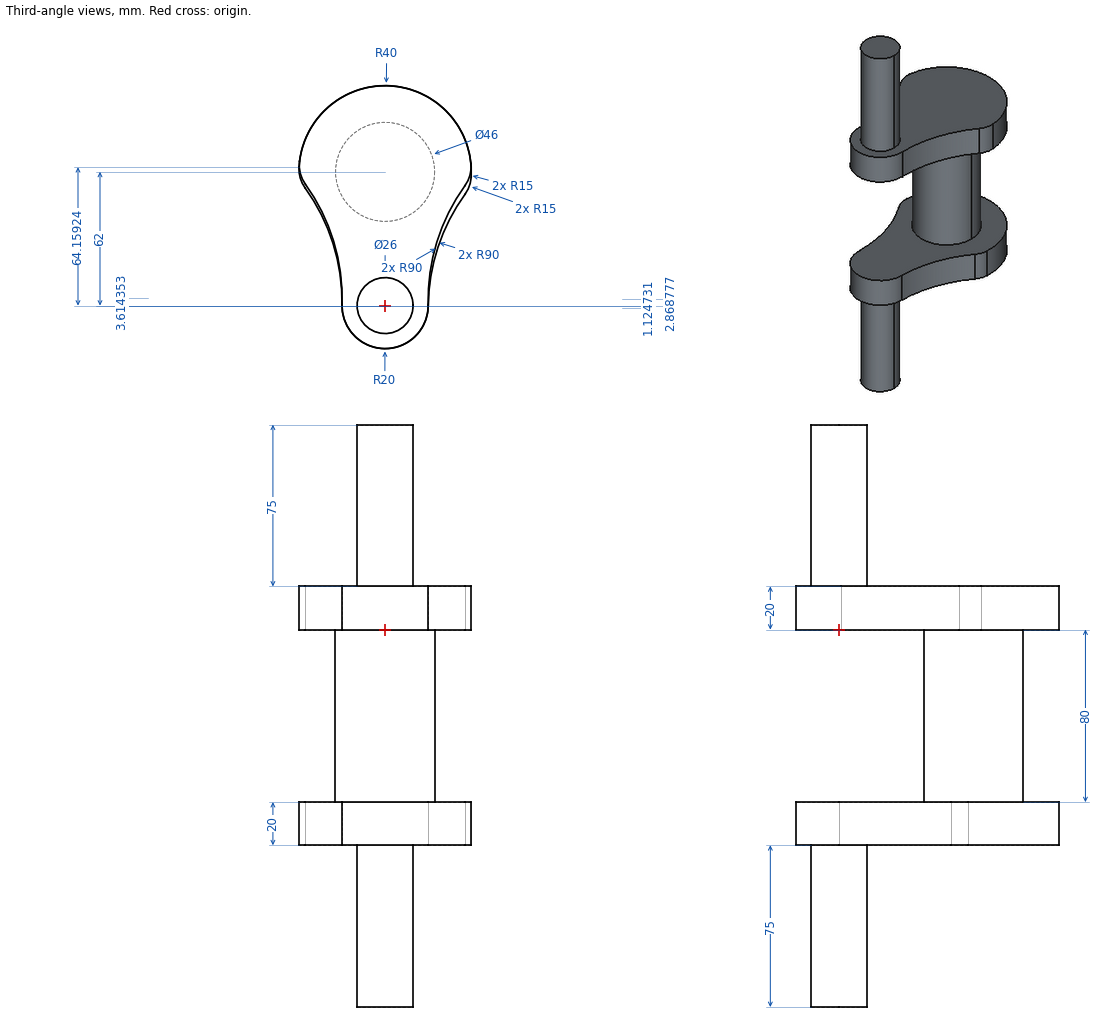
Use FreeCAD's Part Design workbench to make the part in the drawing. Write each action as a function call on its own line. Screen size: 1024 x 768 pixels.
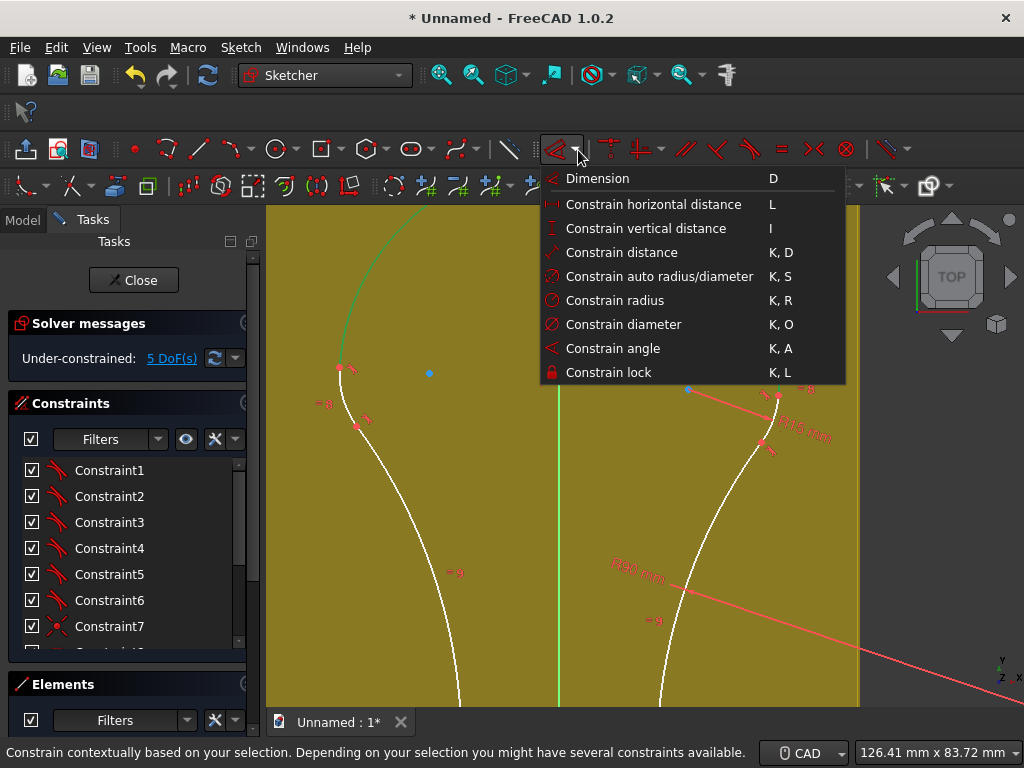
click(693, 300)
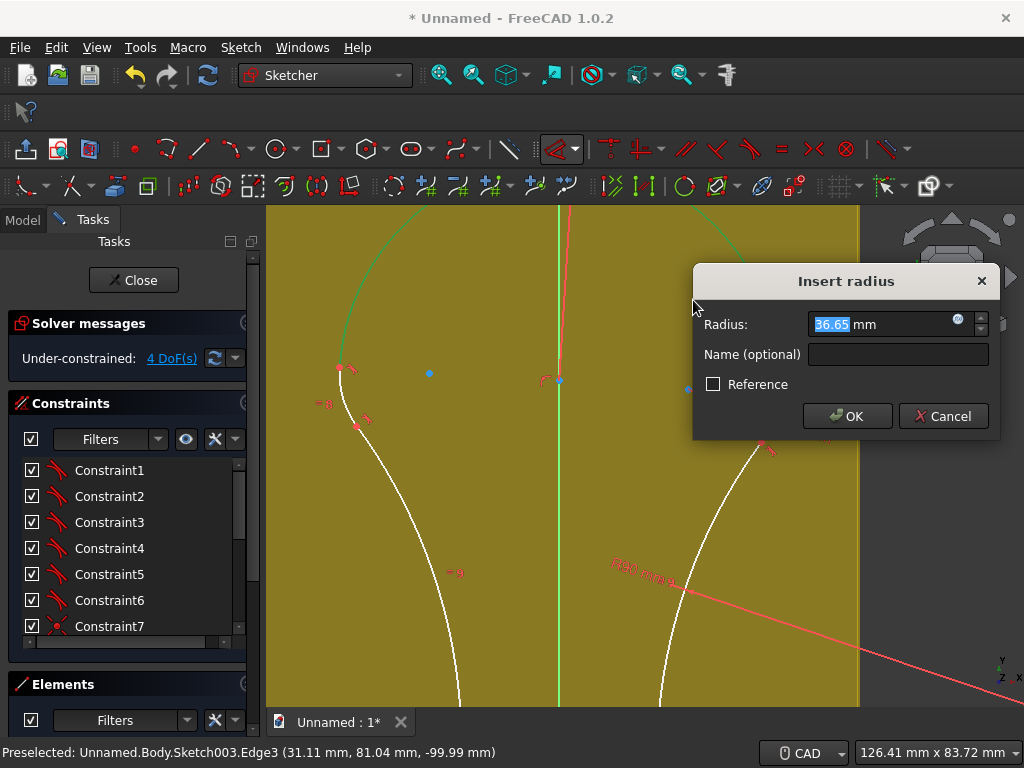
text(40)
key(Return)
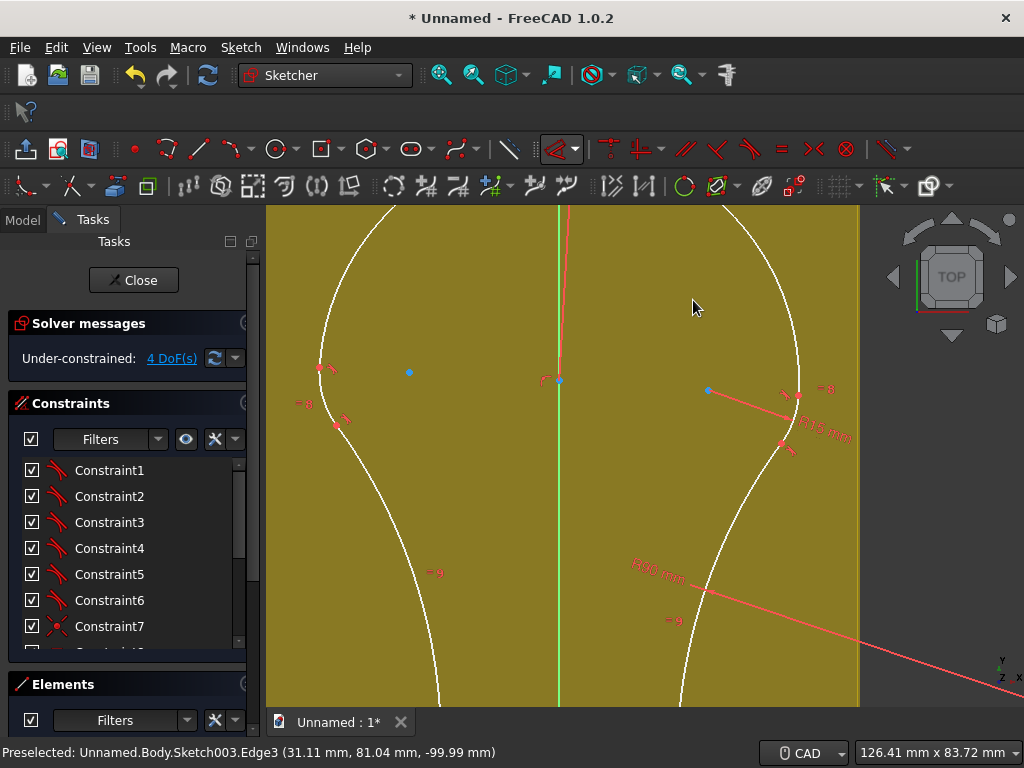
scroll(591, 416, down, 4)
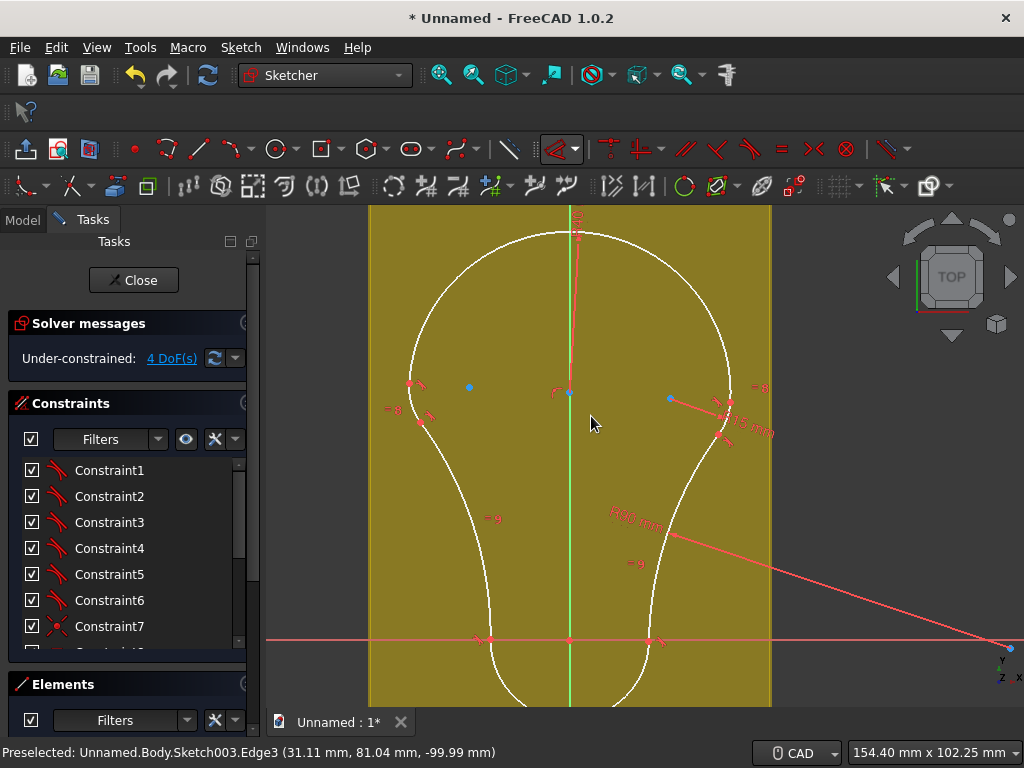
click(545, 609)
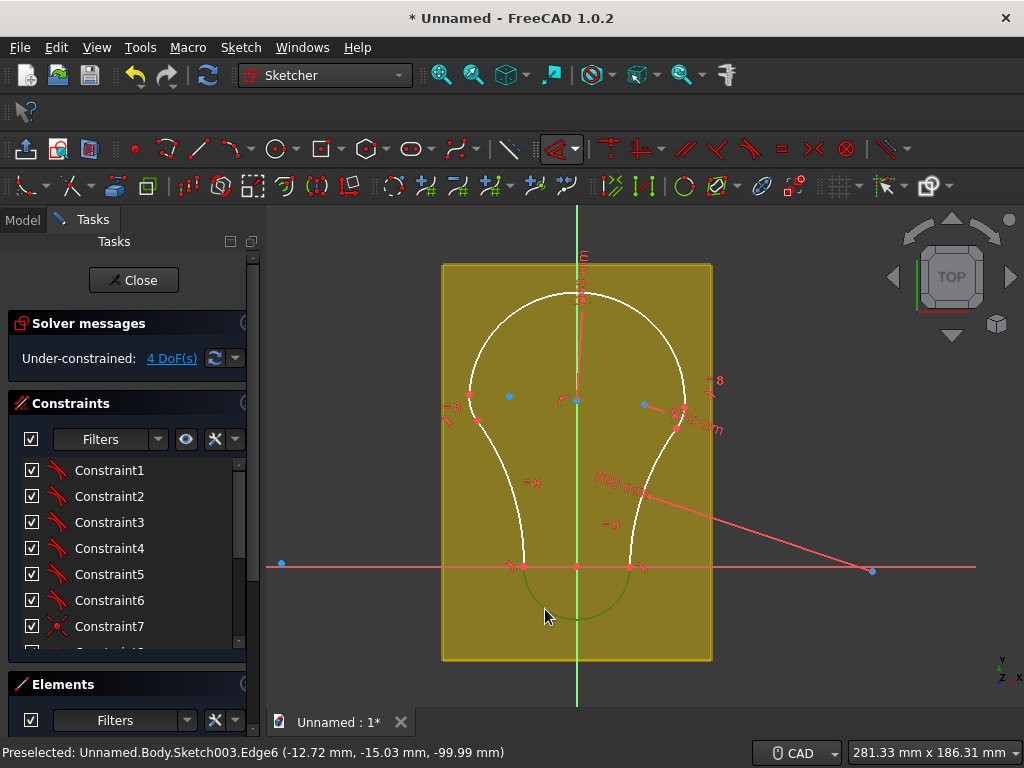
key(k)
key(r)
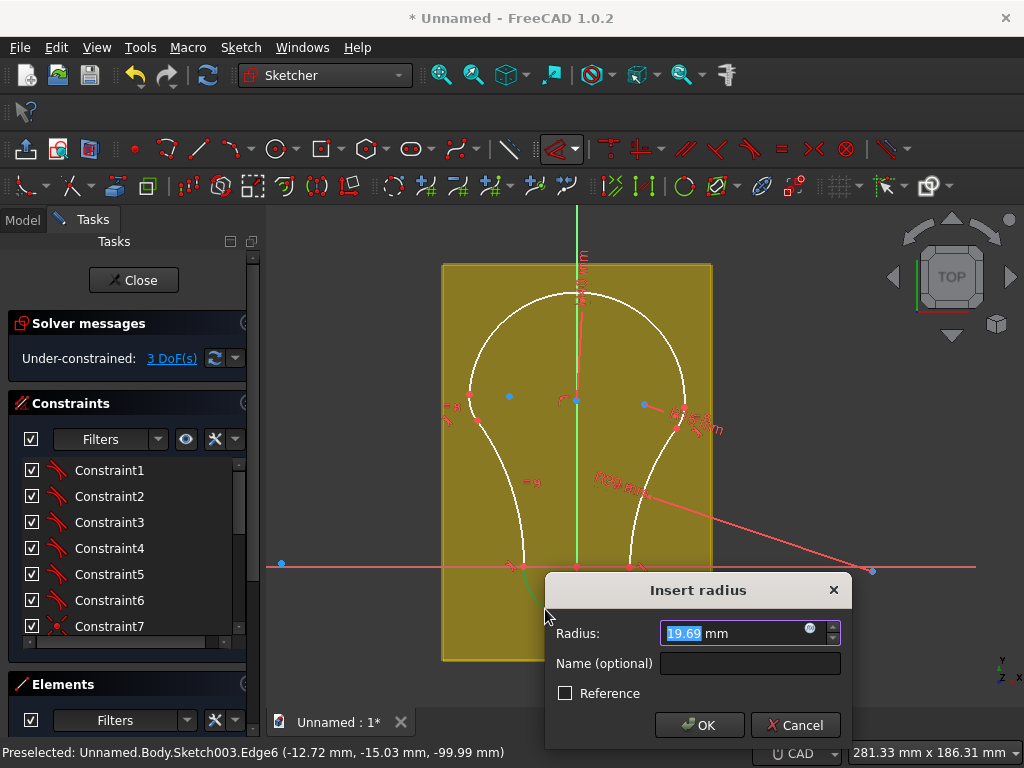
text(20)
key(Return)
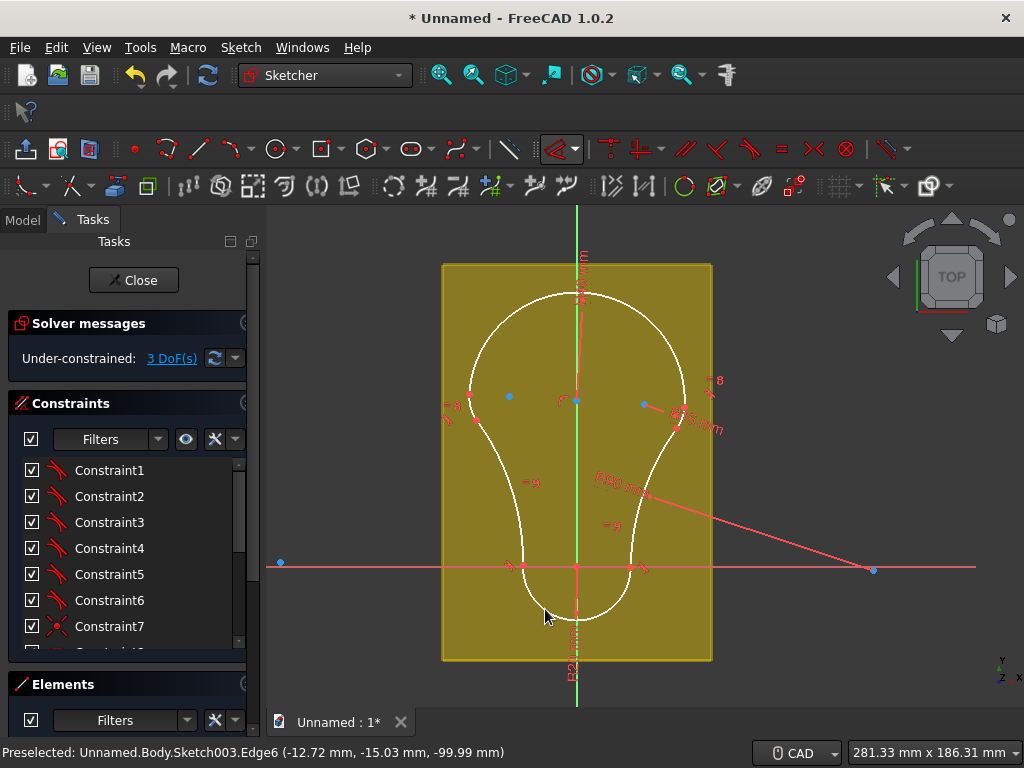
click(577, 400)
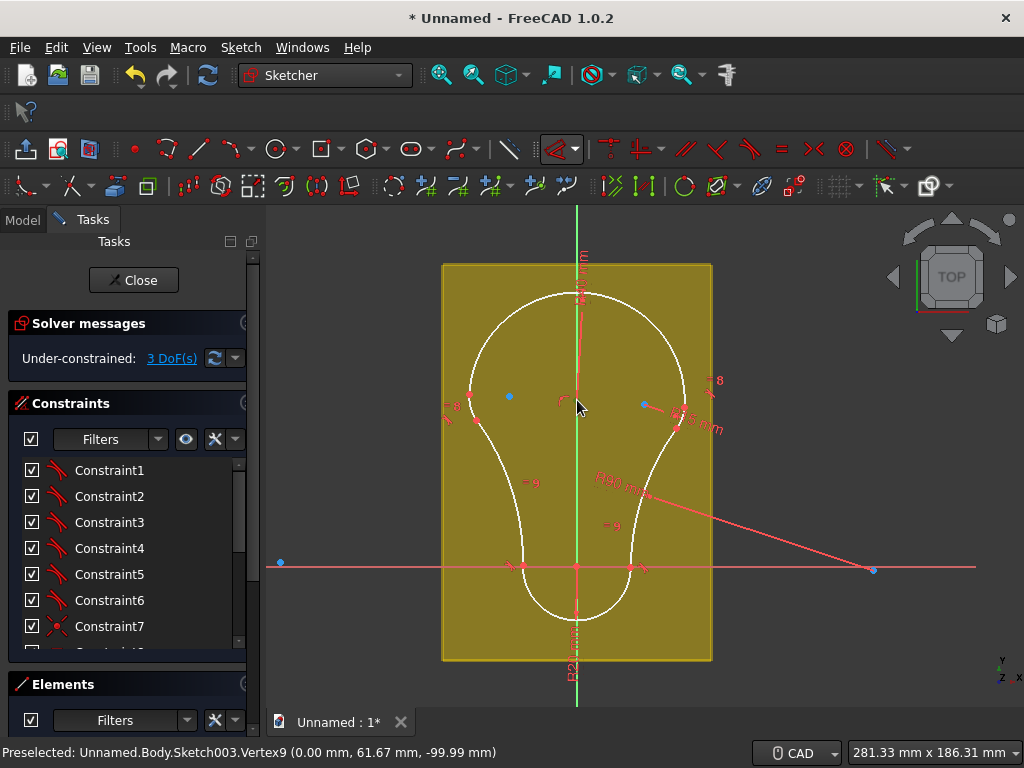
key(i)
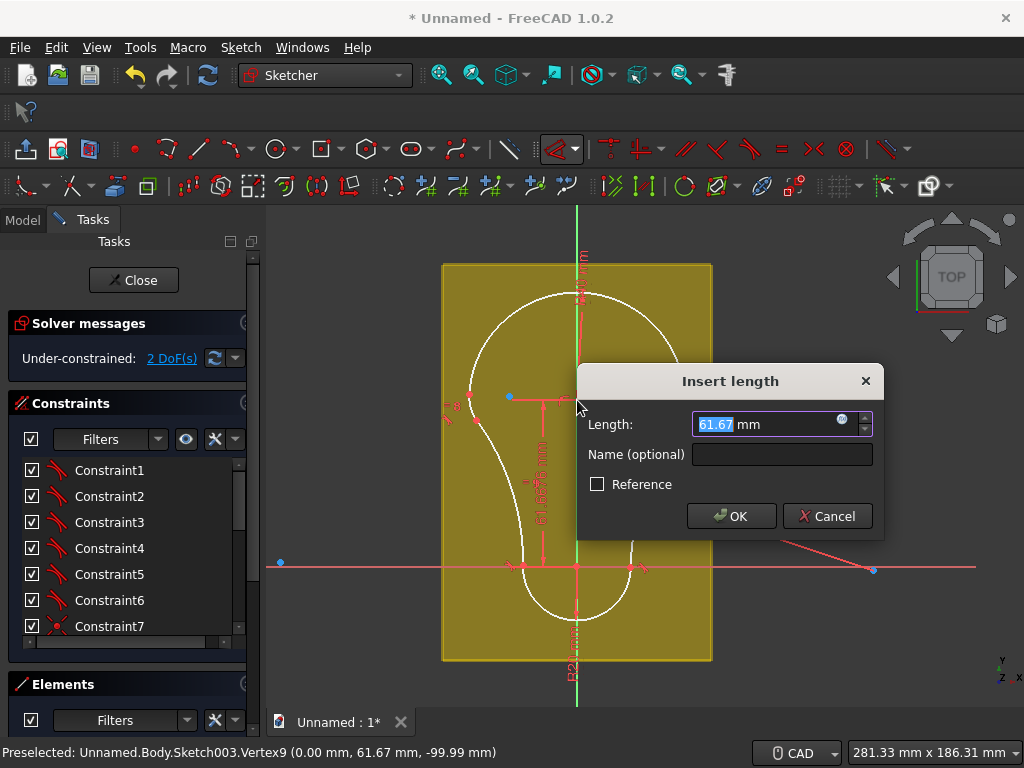
text(62)
key(Return)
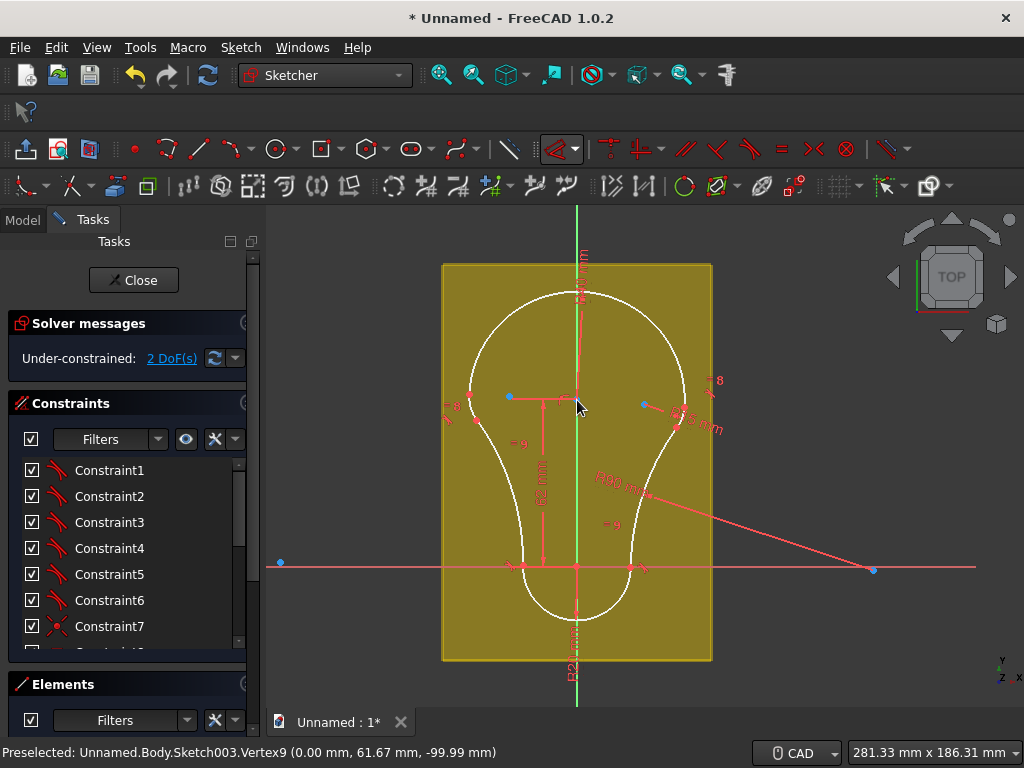
click(469, 395)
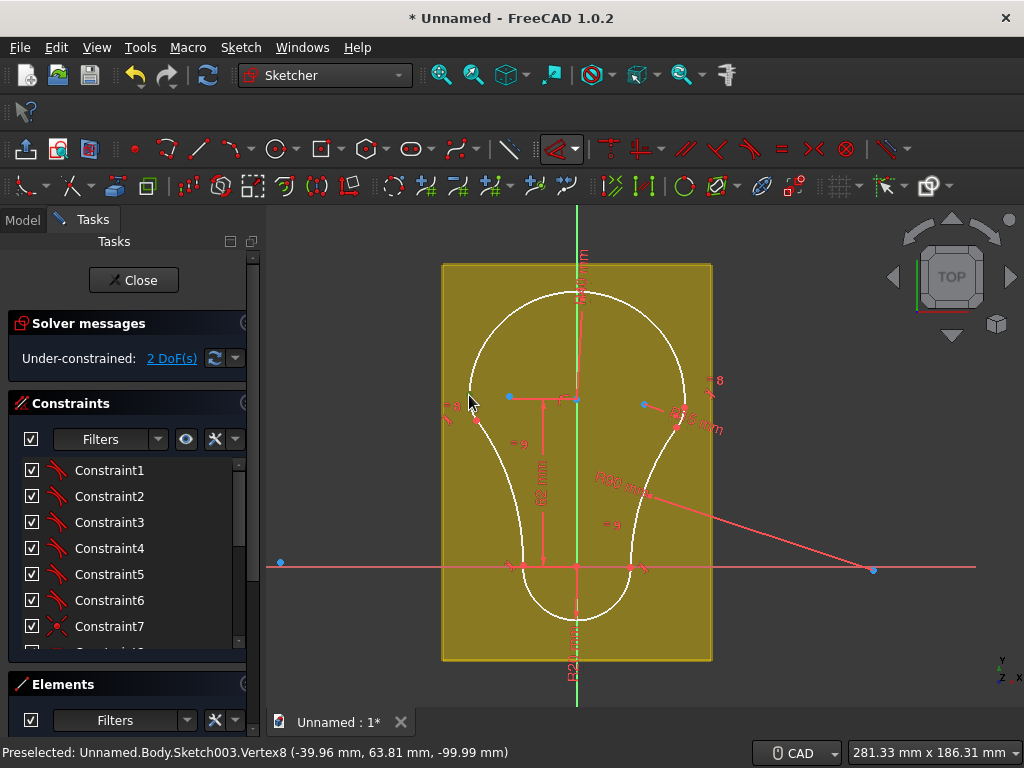
click(578, 150)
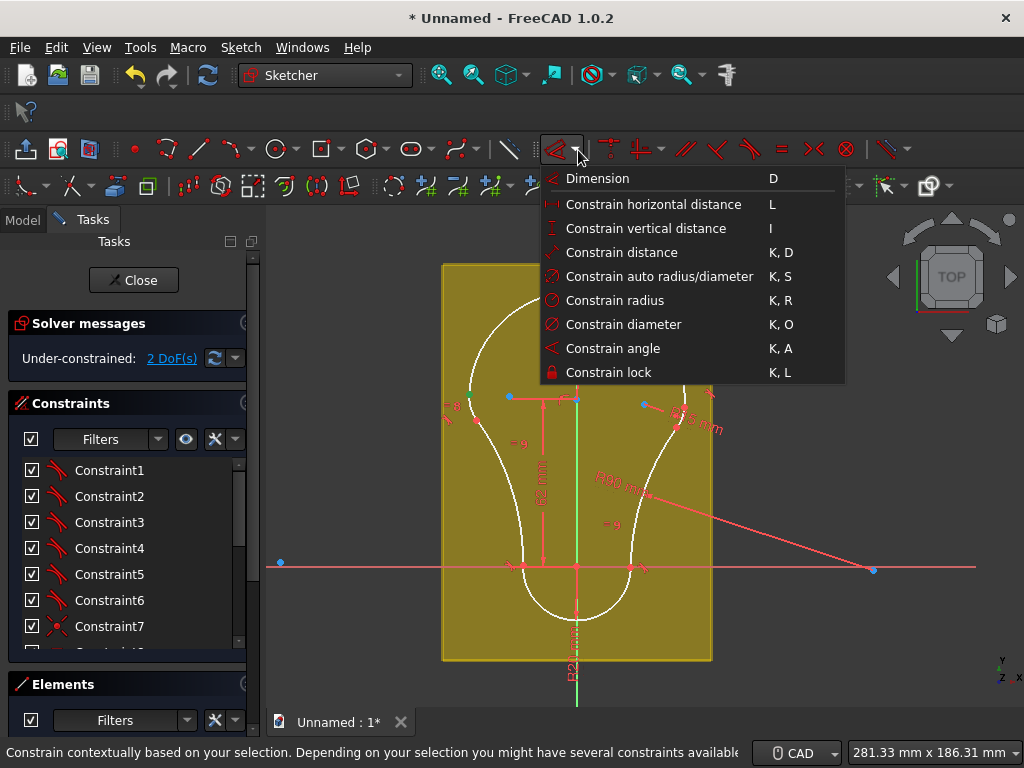
click(693, 228)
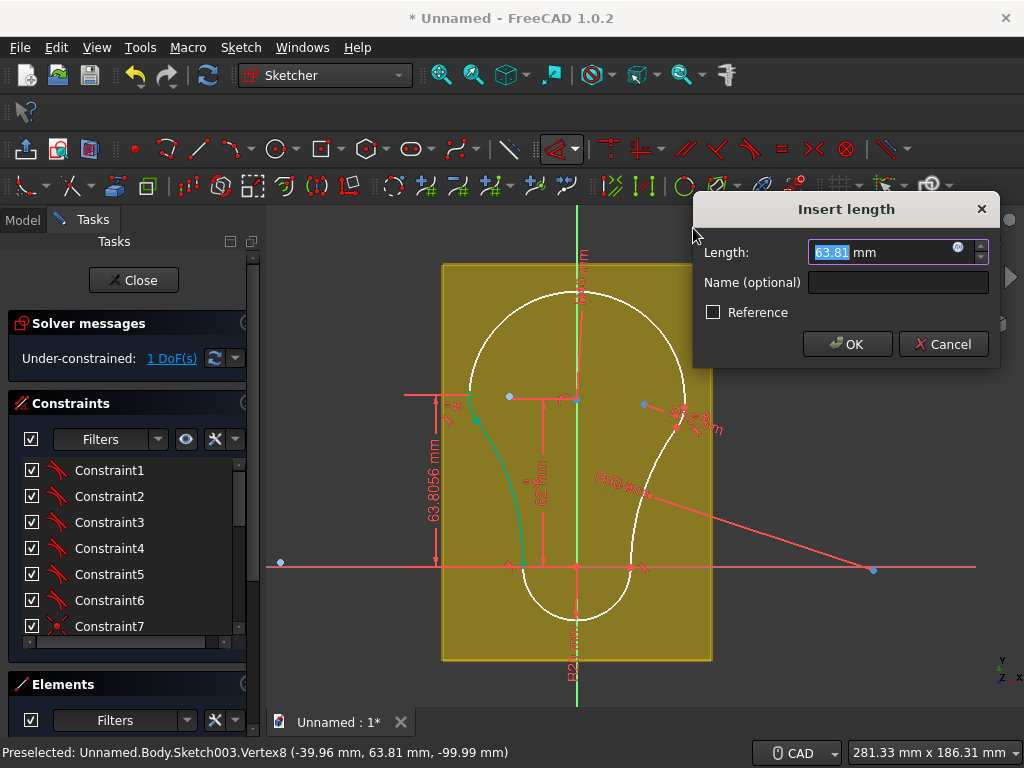
text(64.15924)
key(Return)